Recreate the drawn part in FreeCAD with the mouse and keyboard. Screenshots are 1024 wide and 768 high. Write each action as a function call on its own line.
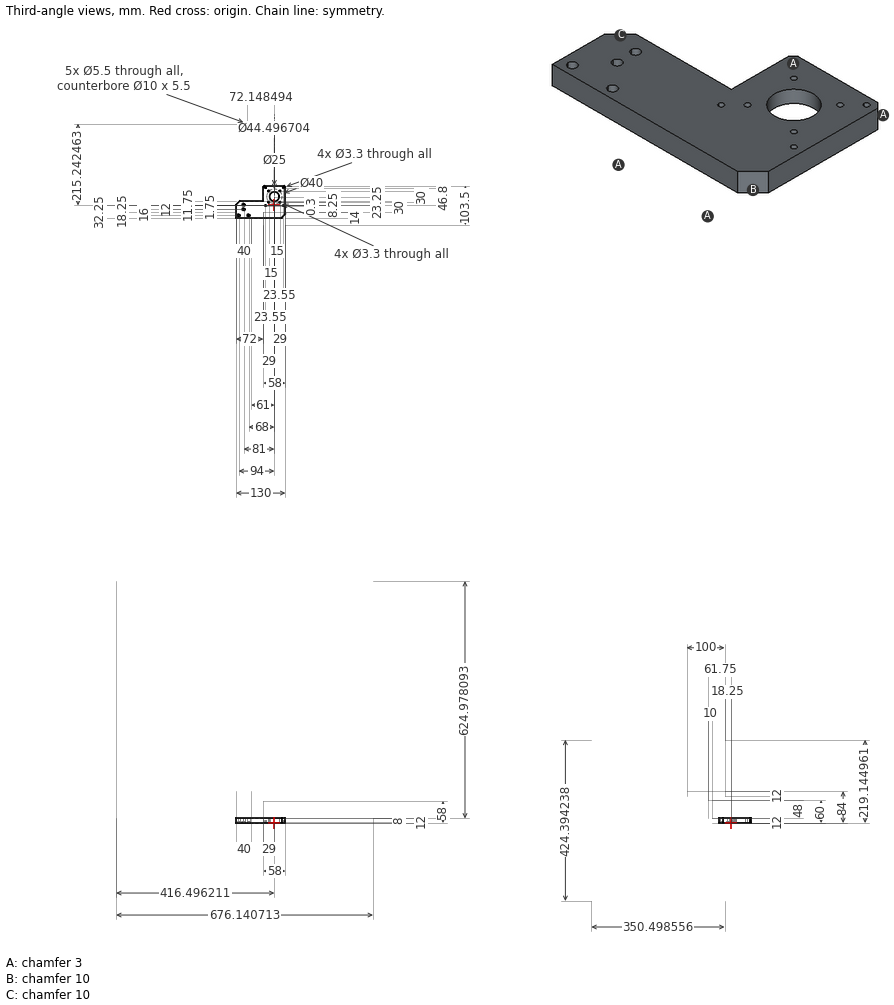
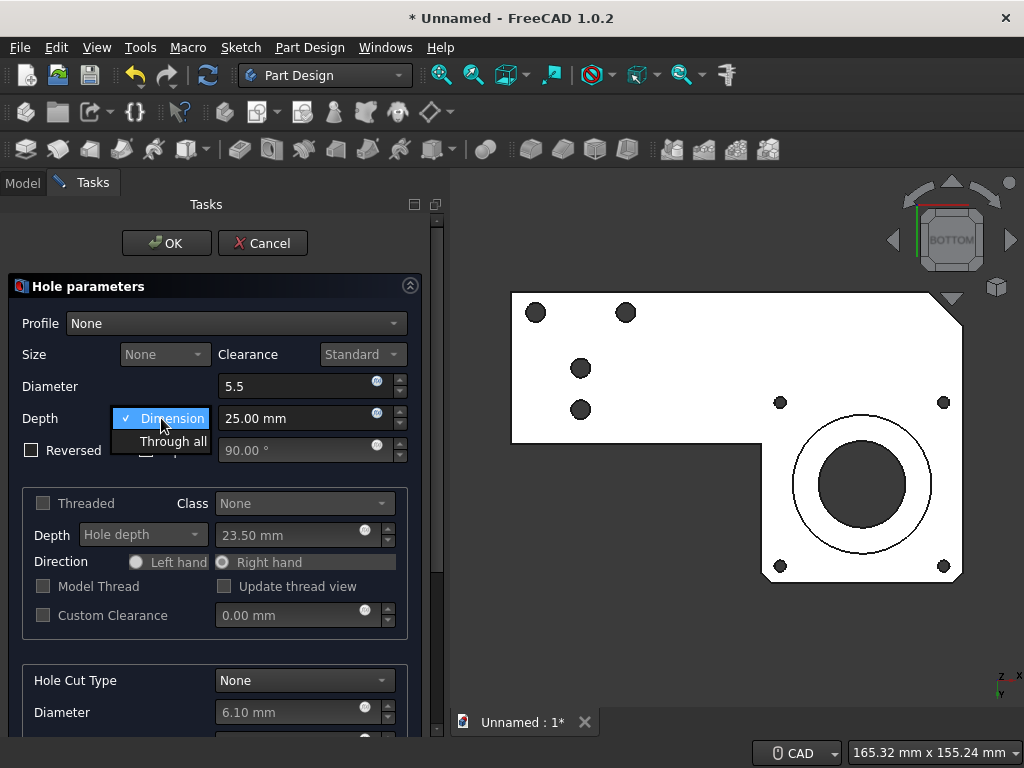
click(160, 442)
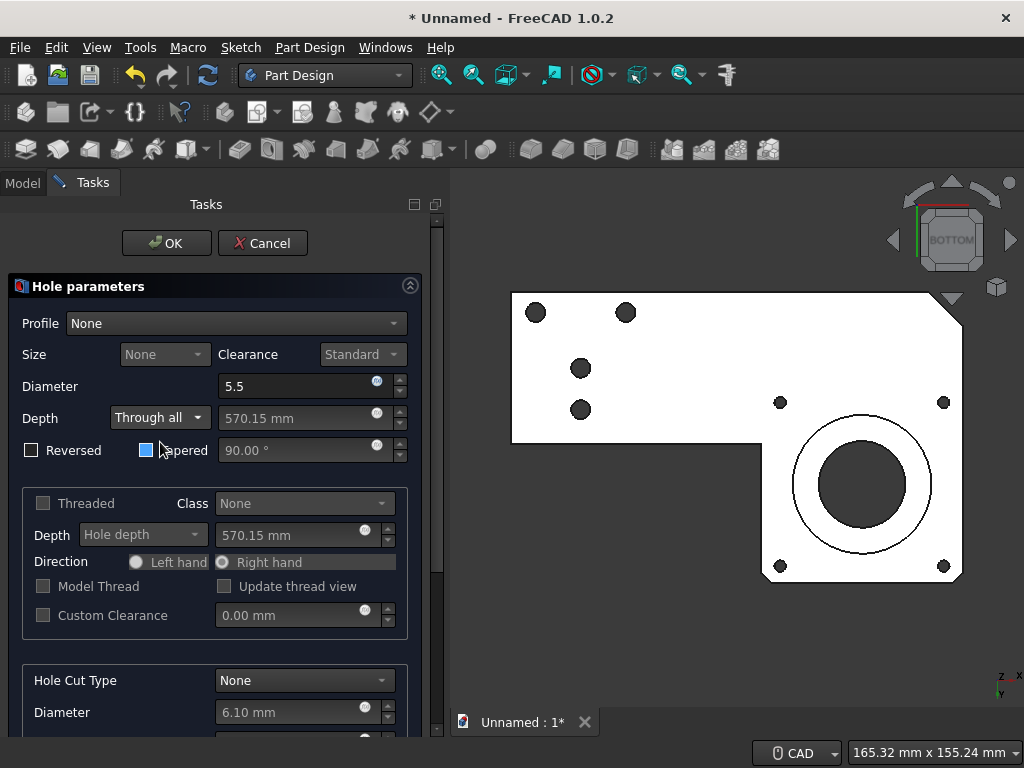
click(306, 680)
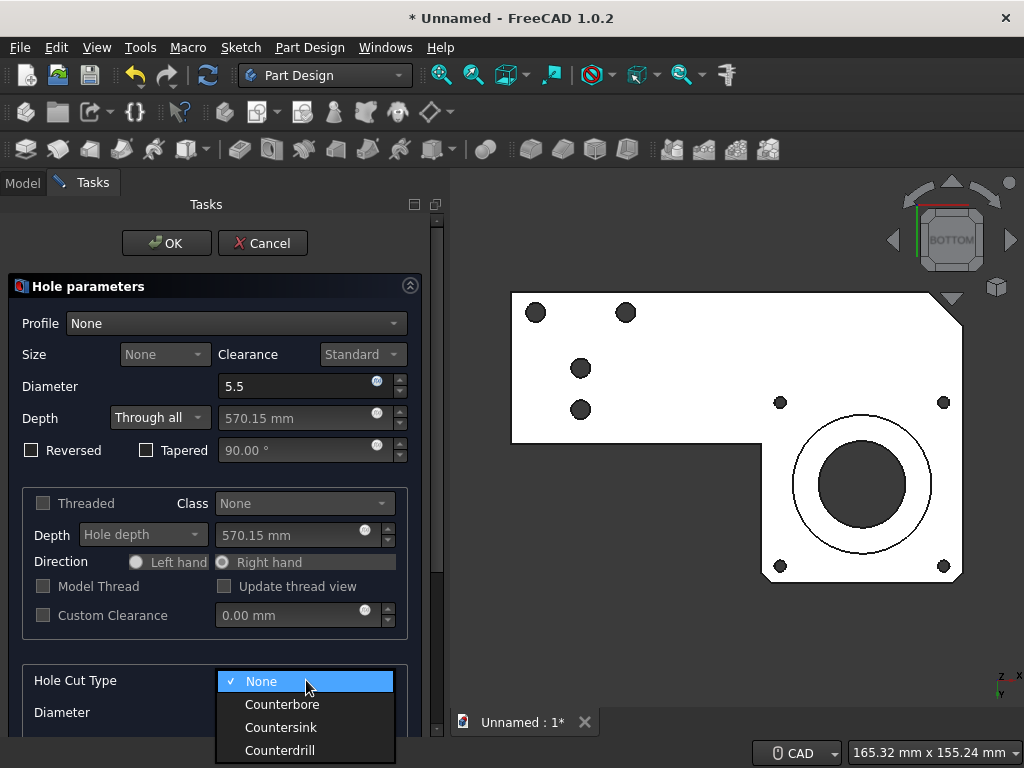
click(304, 704)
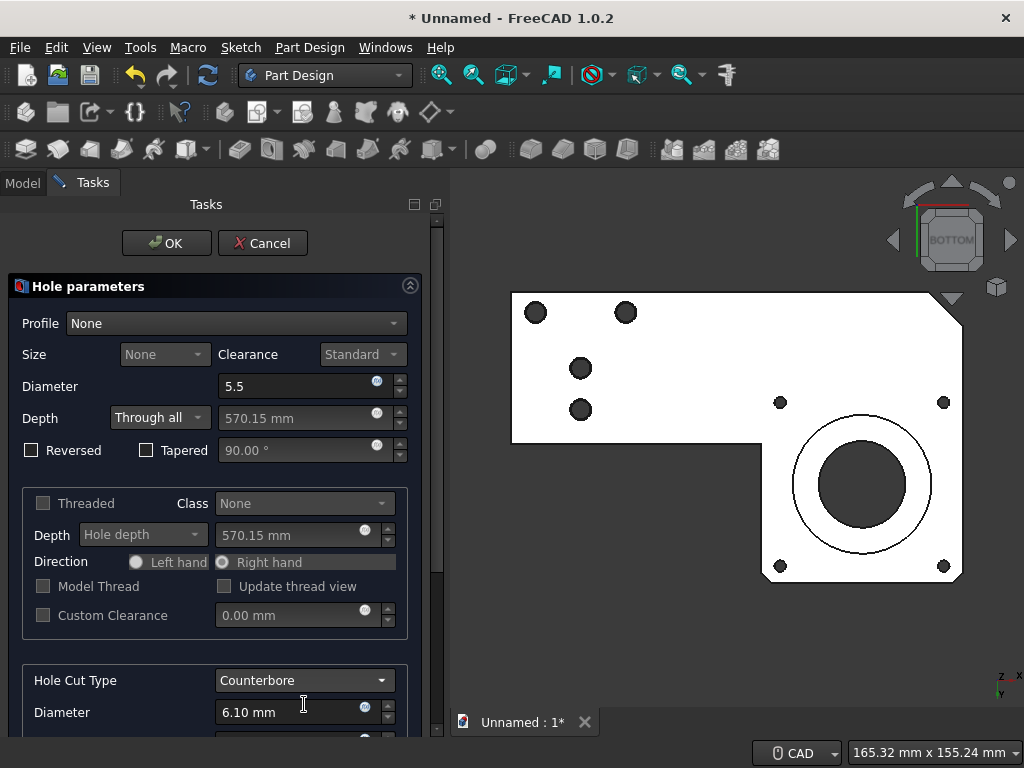
triple_click(298, 712)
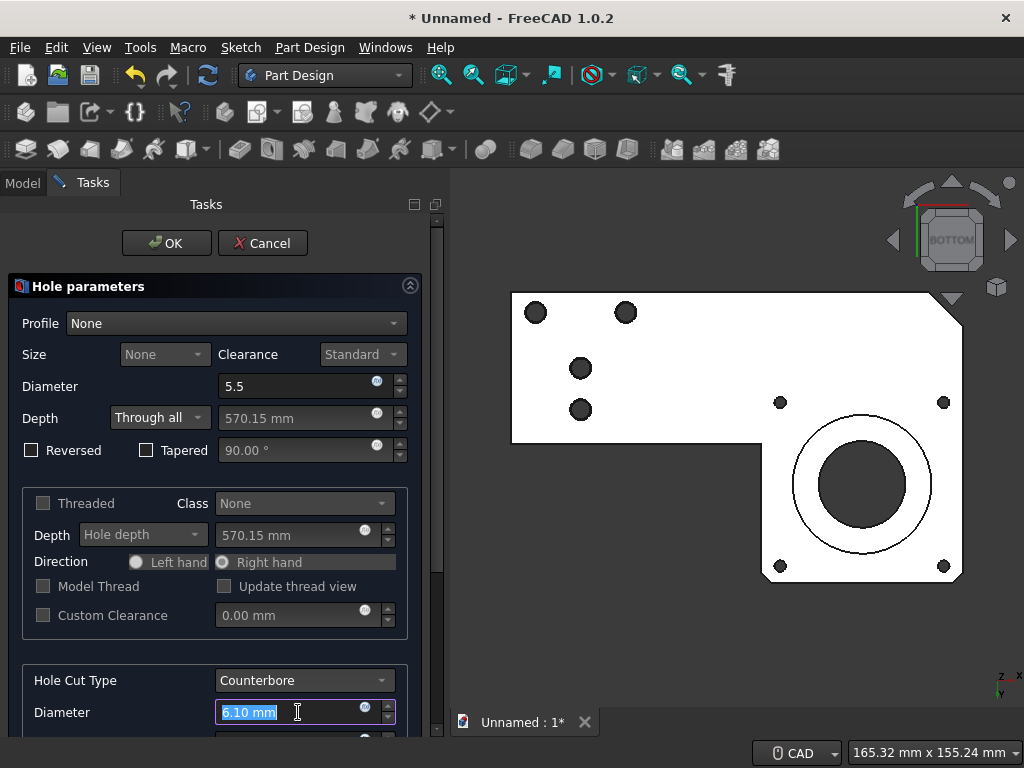
text(10)
key(Tab)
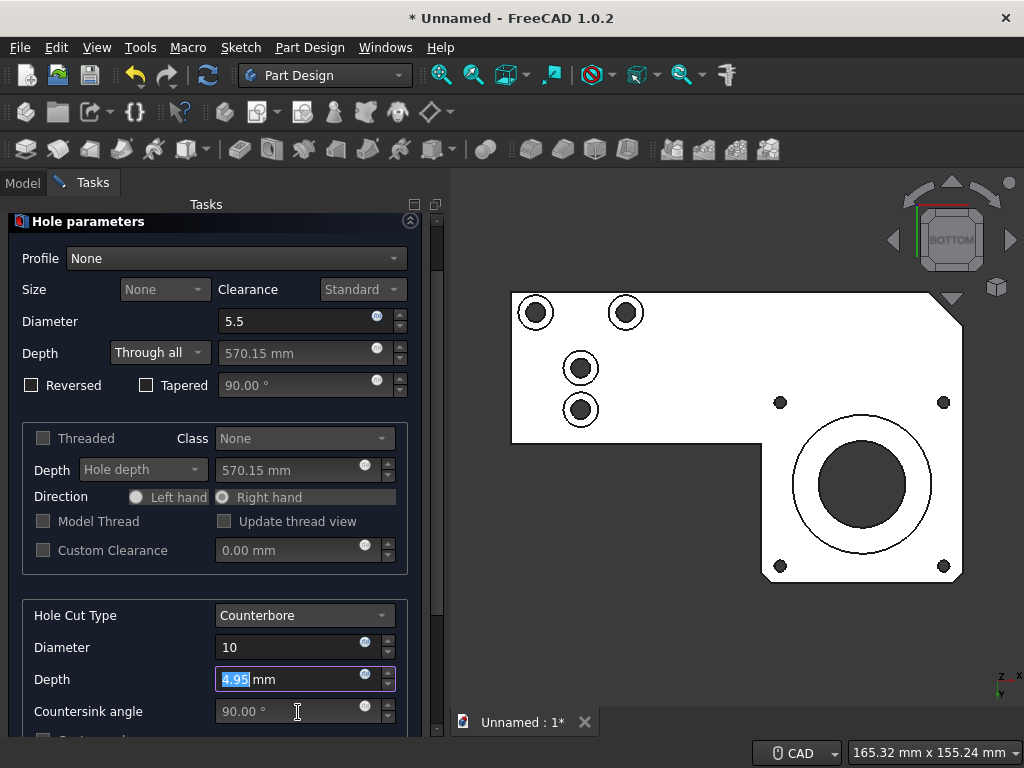
text(5.5)
key(Tab)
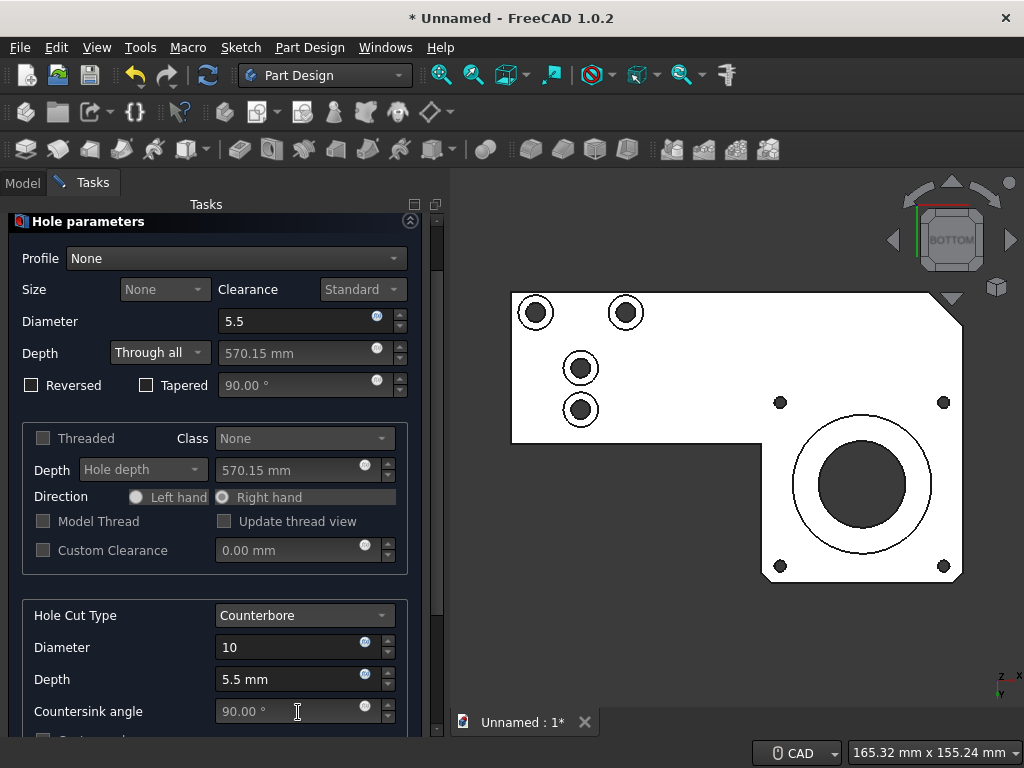
scroll(437, 475, up, 2)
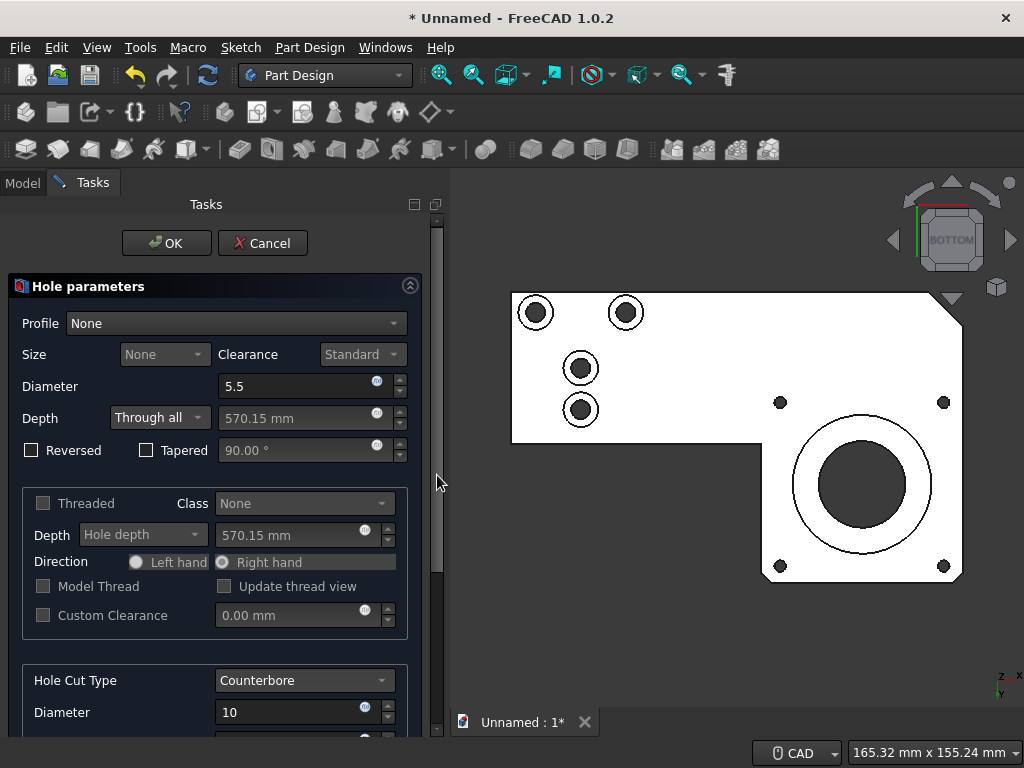
click(167, 243)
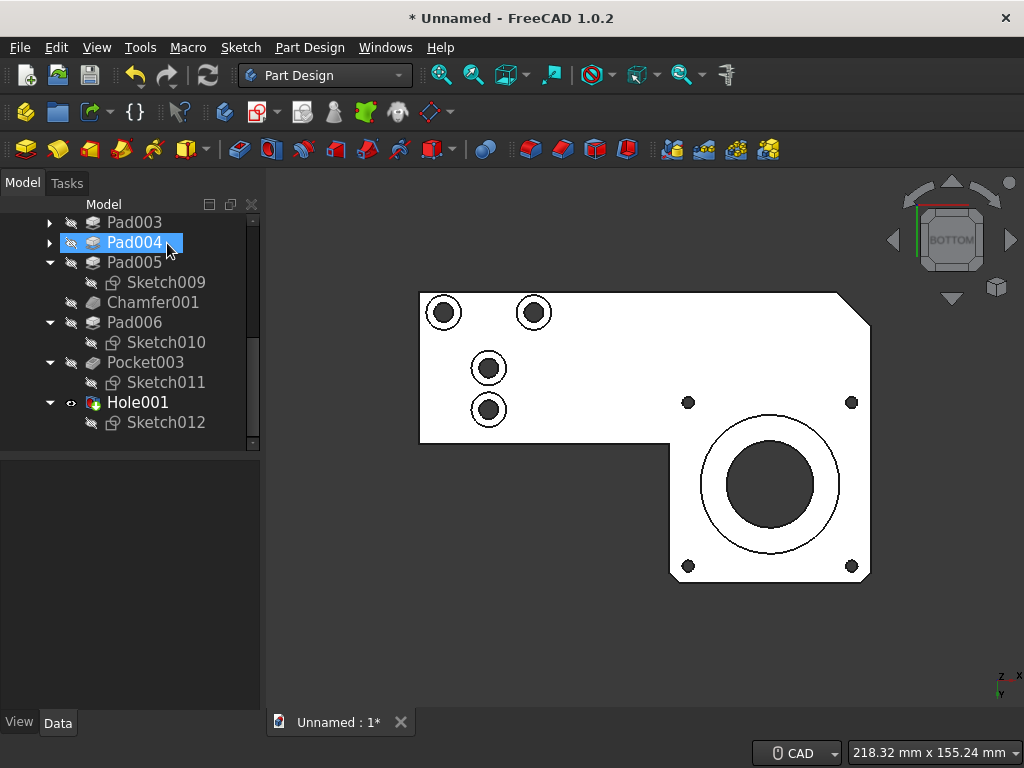
key(0)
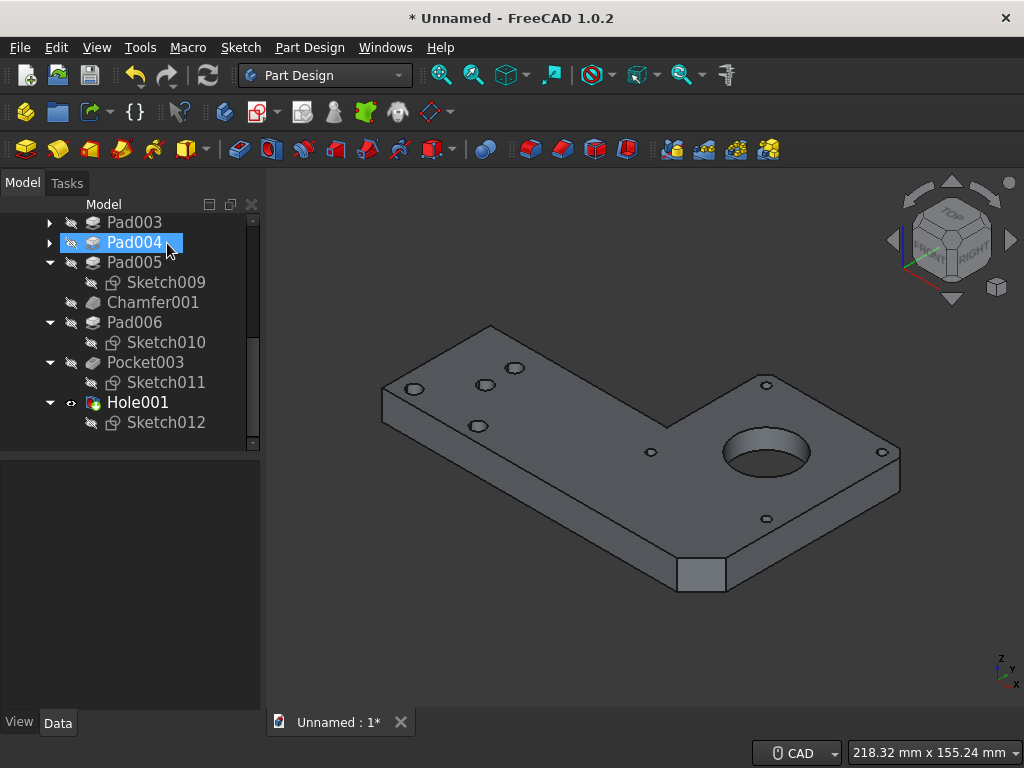
key(2)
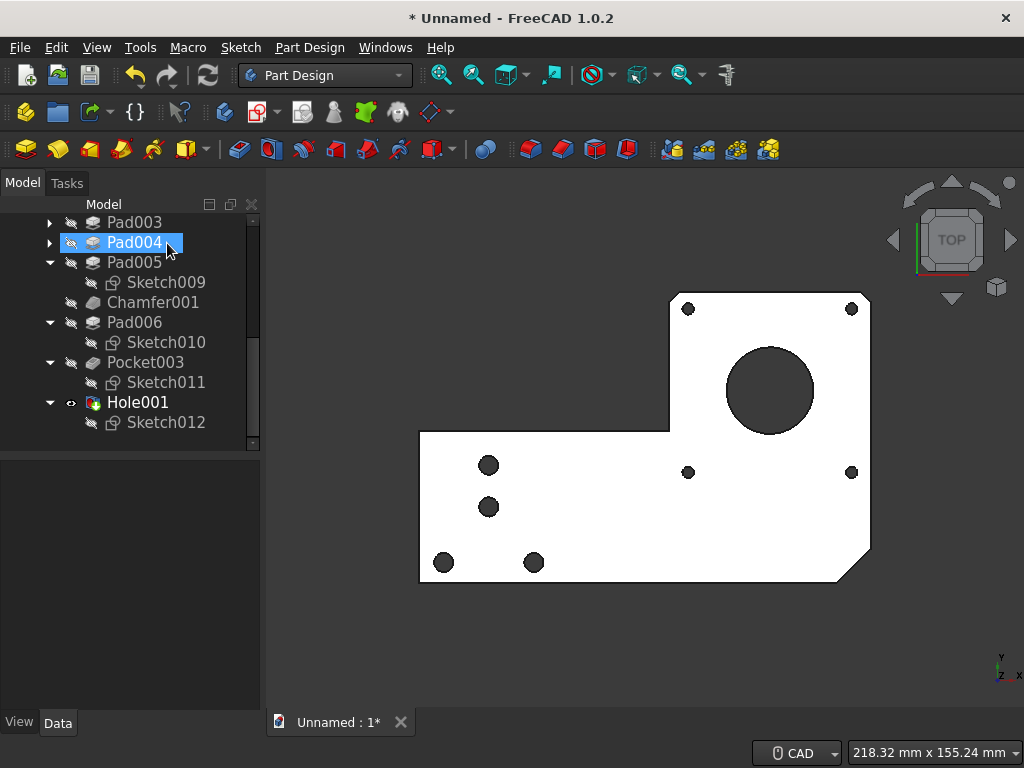
key(1)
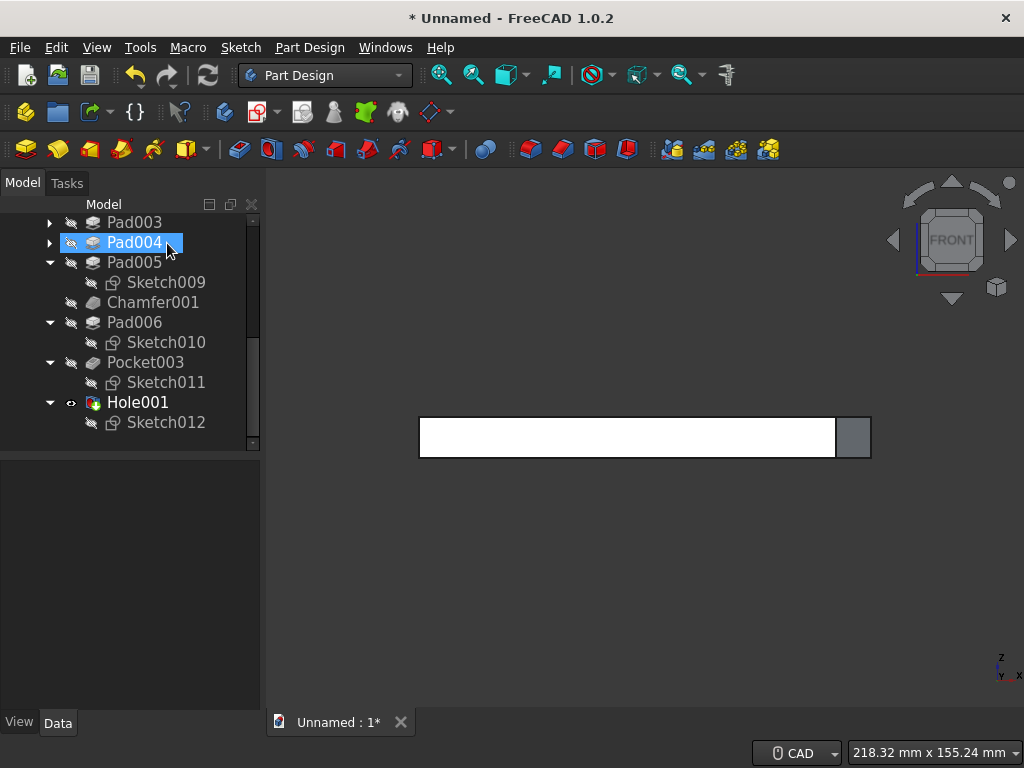
key(3)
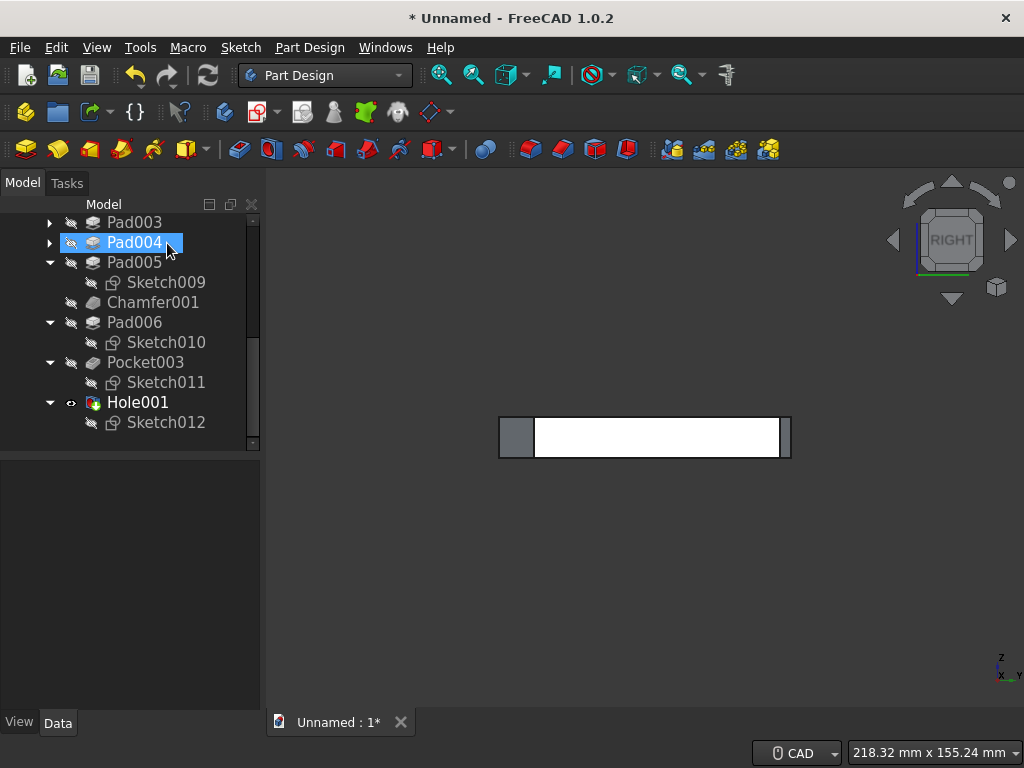
key(v)
key(f)